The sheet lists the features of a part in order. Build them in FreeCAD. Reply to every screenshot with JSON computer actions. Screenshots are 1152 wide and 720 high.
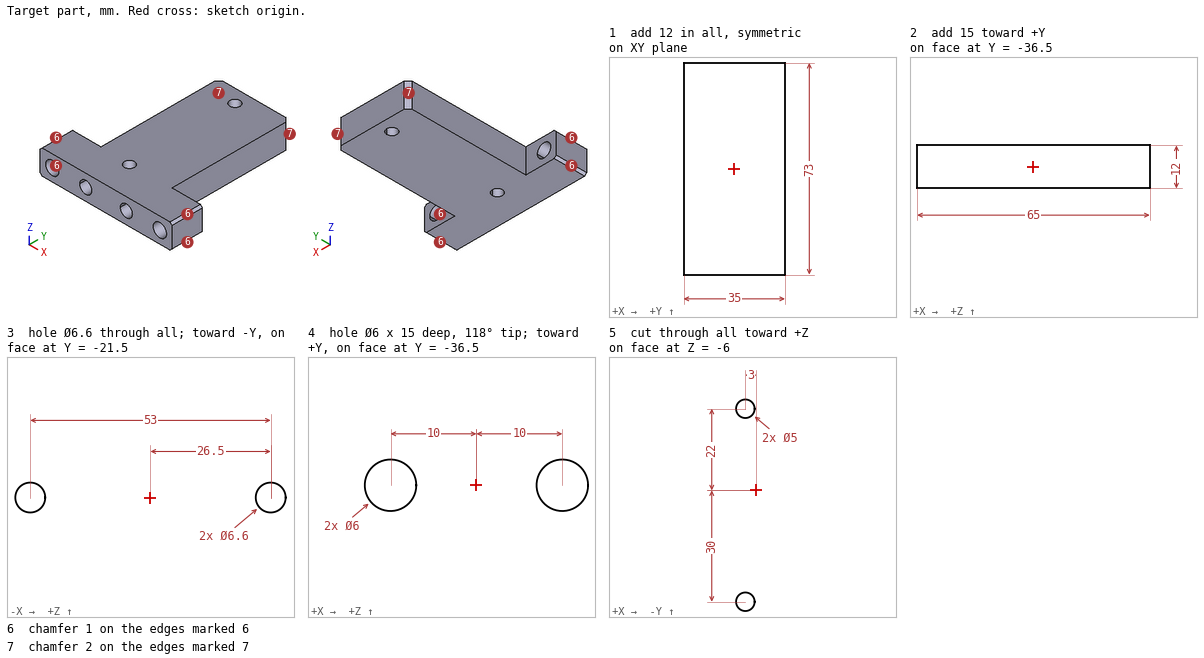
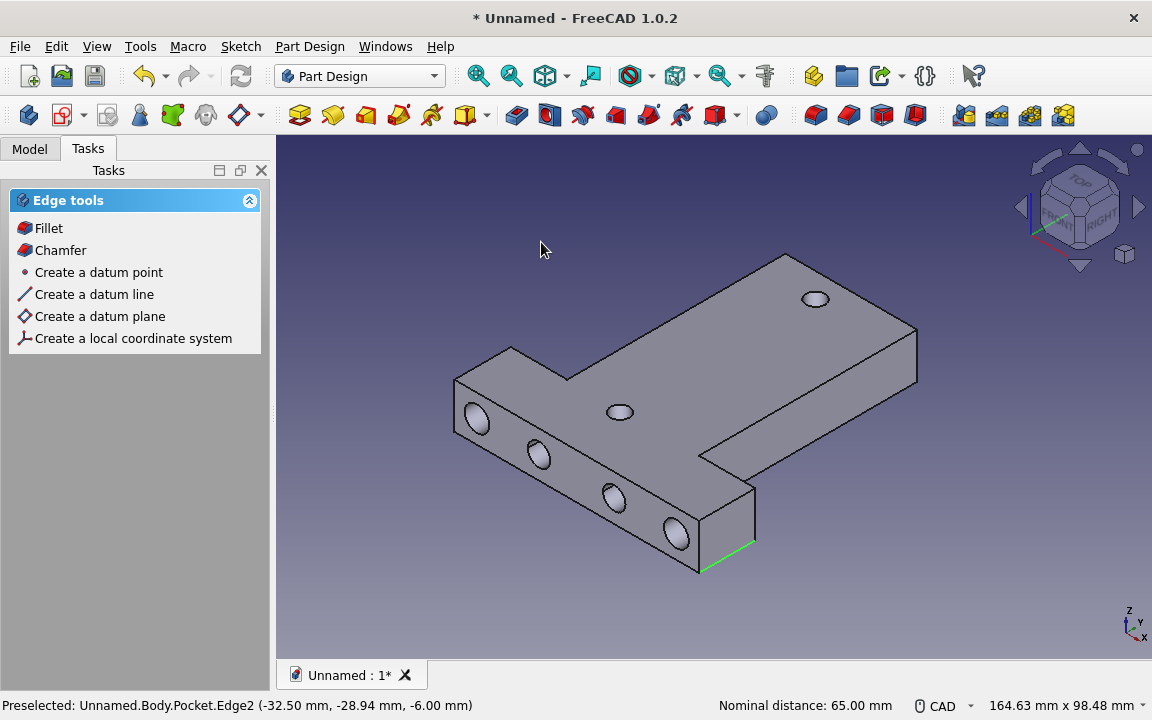
{"action": "left_click", "coordinate": [727, 504], "text": "ctrl"}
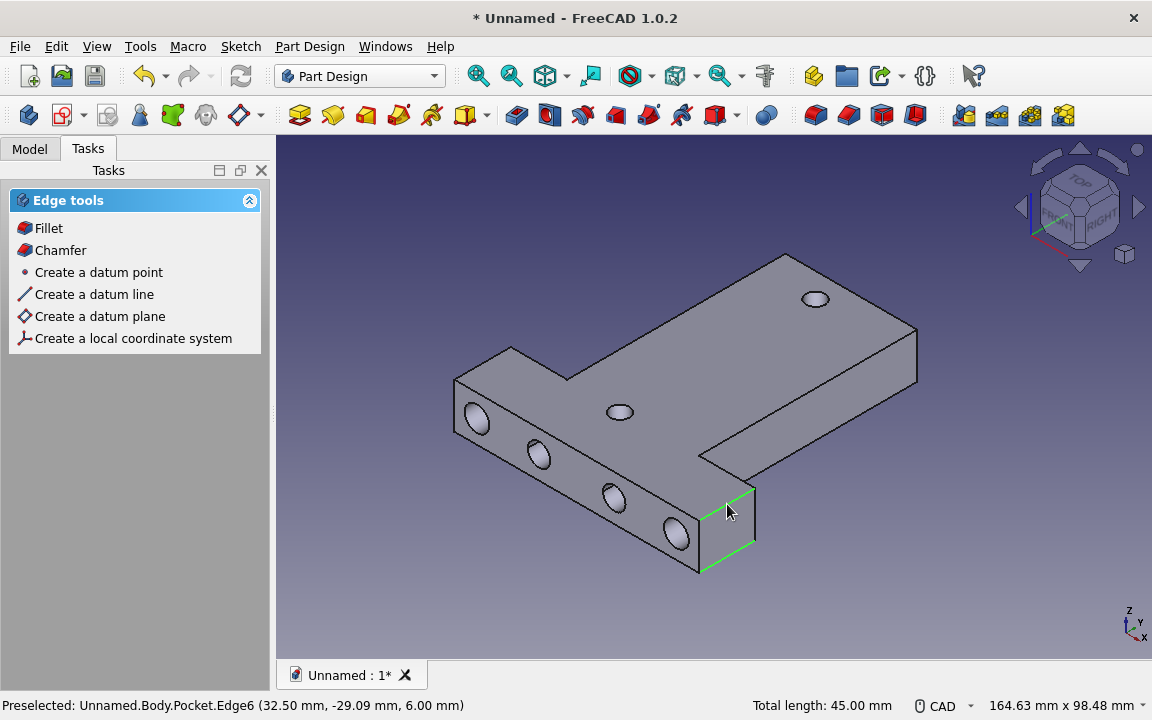
{"action": "key", "text": "2"}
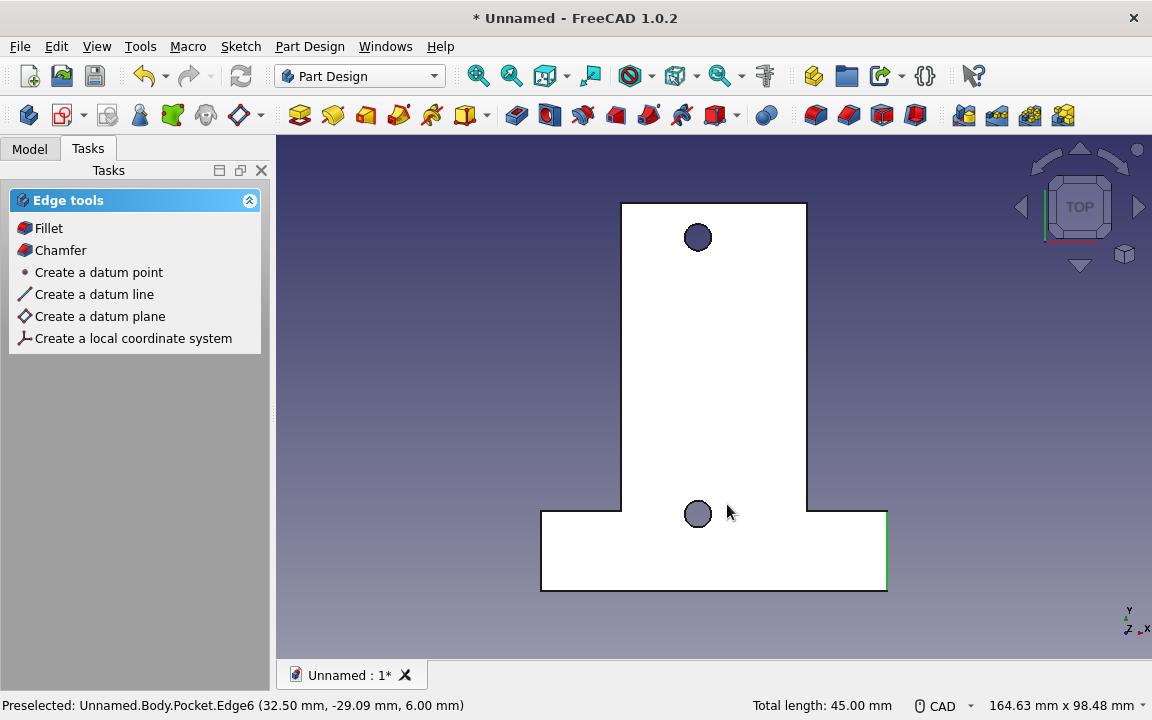
{"action": "left_click", "coordinate": [541, 550], "text": "ctrl"}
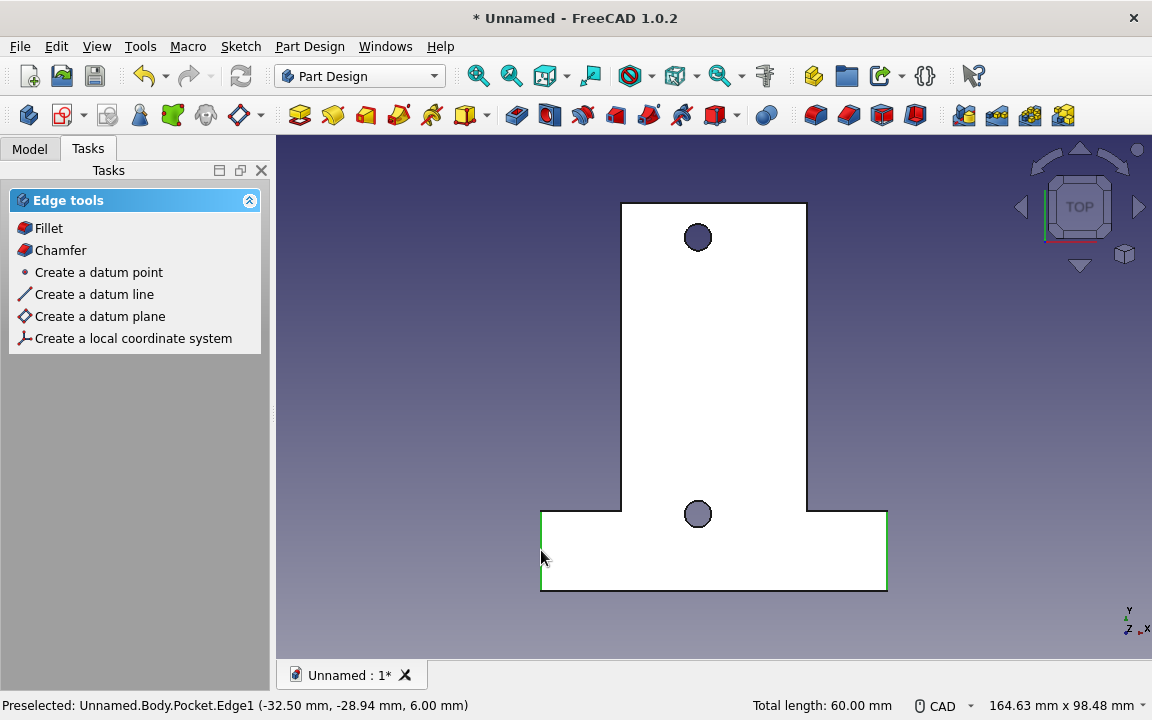
{"action": "left_click", "coordinate": [849, 116]}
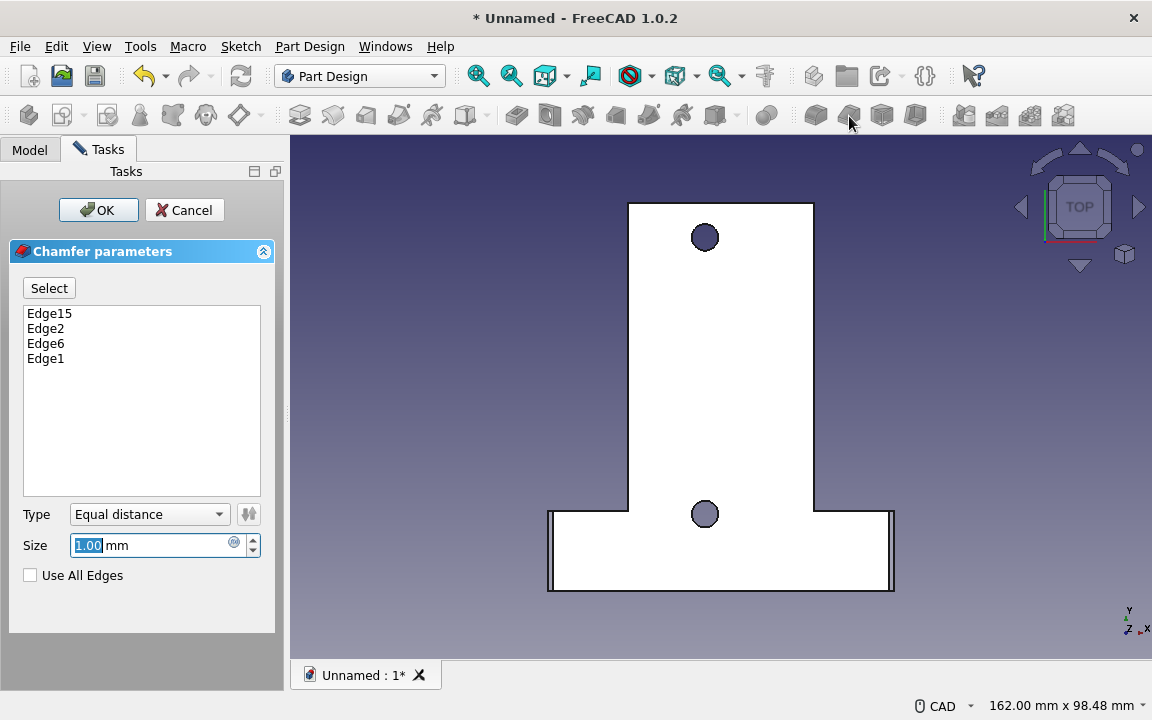
{"action": "type", "text": "1"}
{"action": "key", "text": "Tab"}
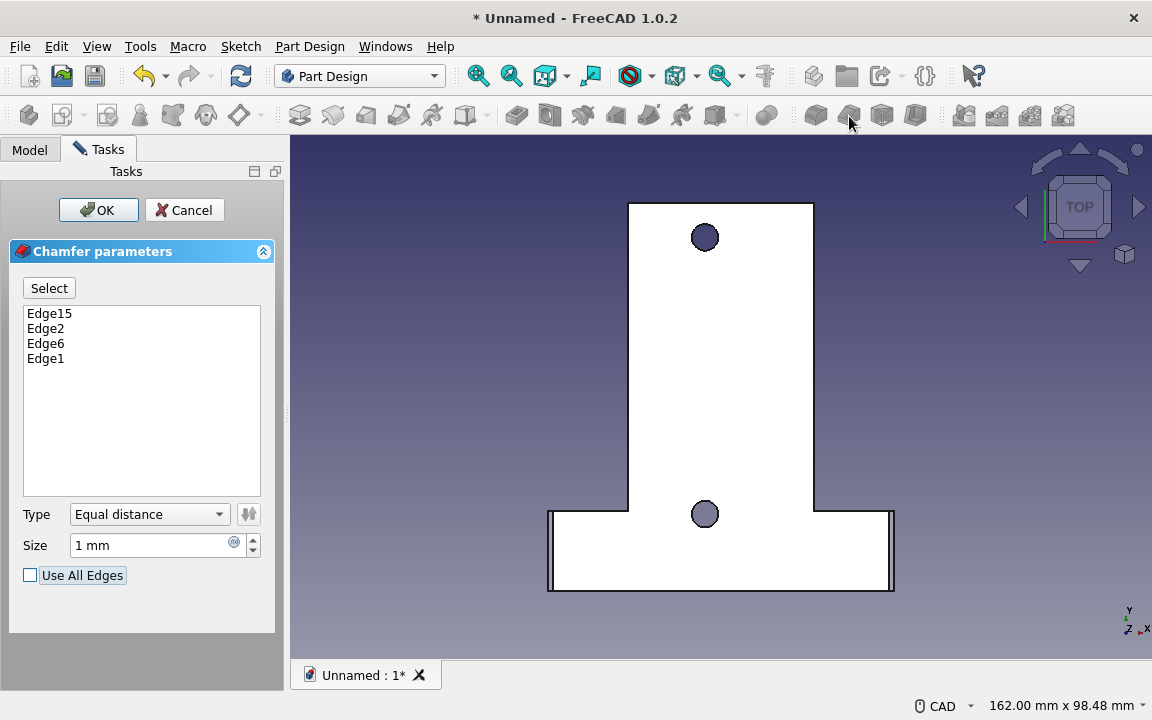
{"action": "left_click", "coordinate": [99, 210]}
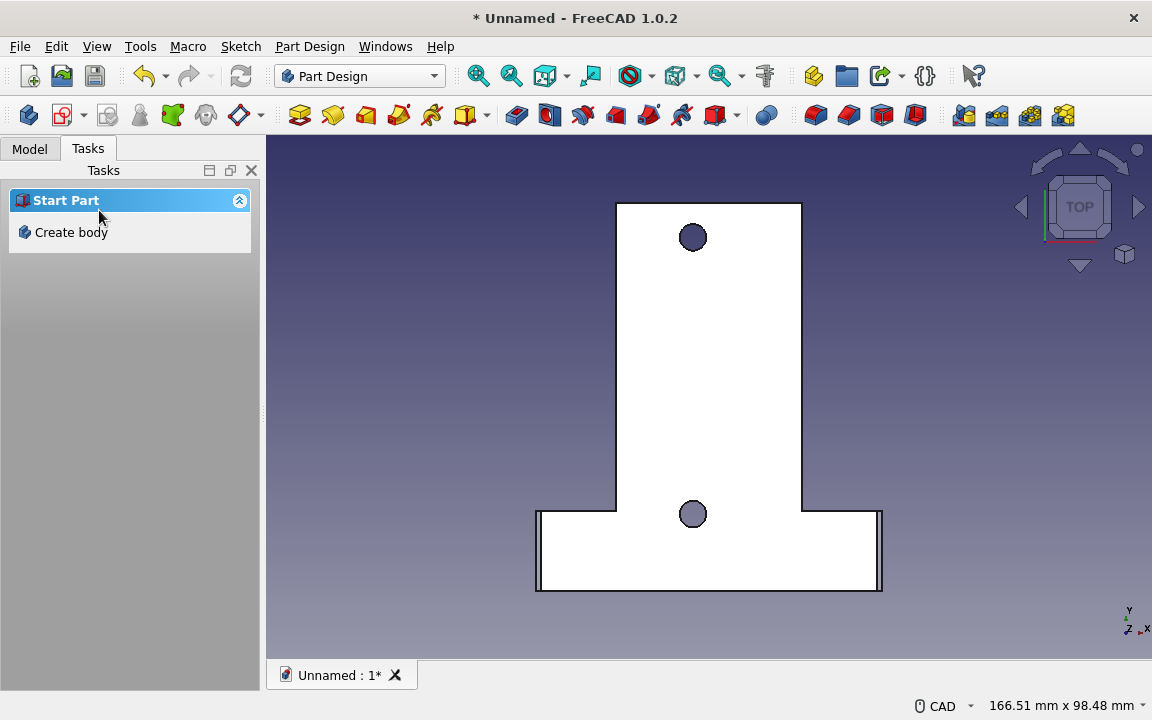
{"action": "key", "text": "0"}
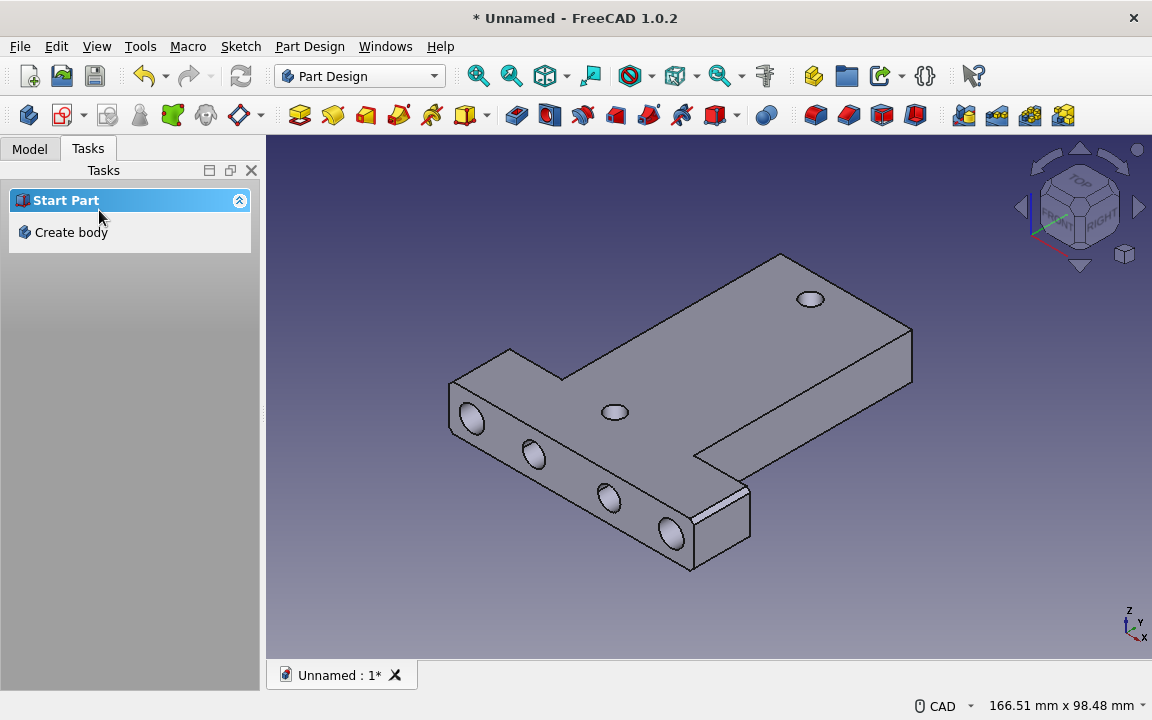
{"action": "key", "text": "2"}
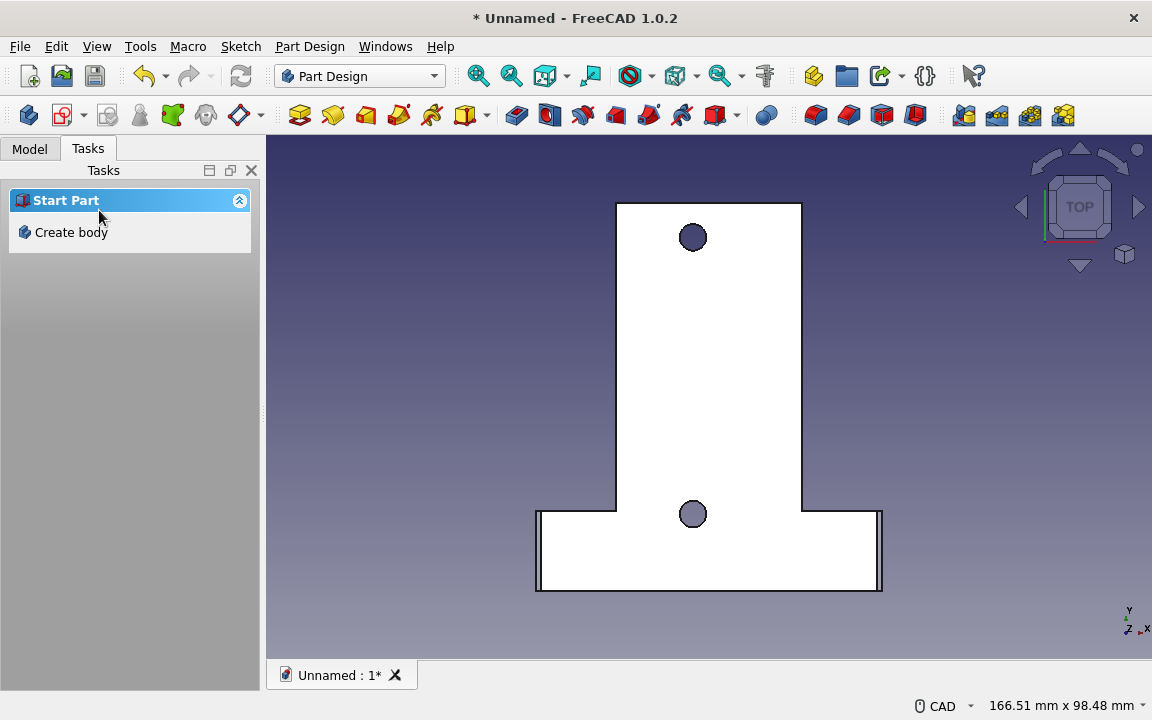
{"action": "key", "text": "1"}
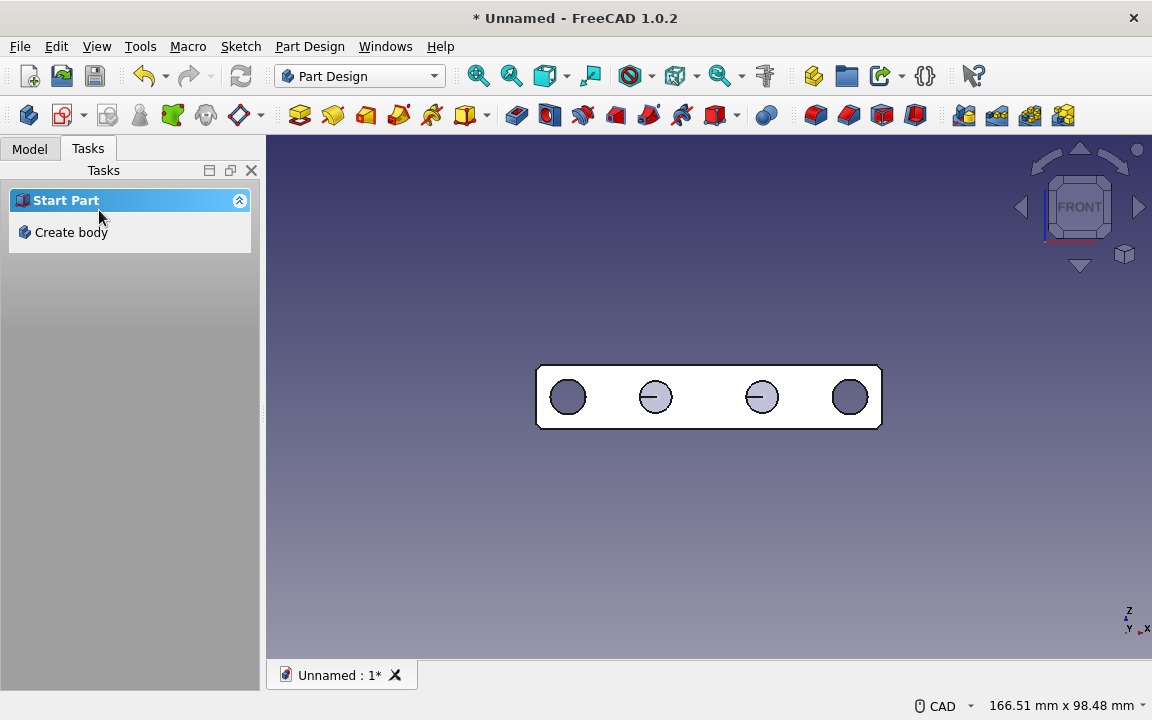
{"action": "left_click", "coordinate": [479, 76]}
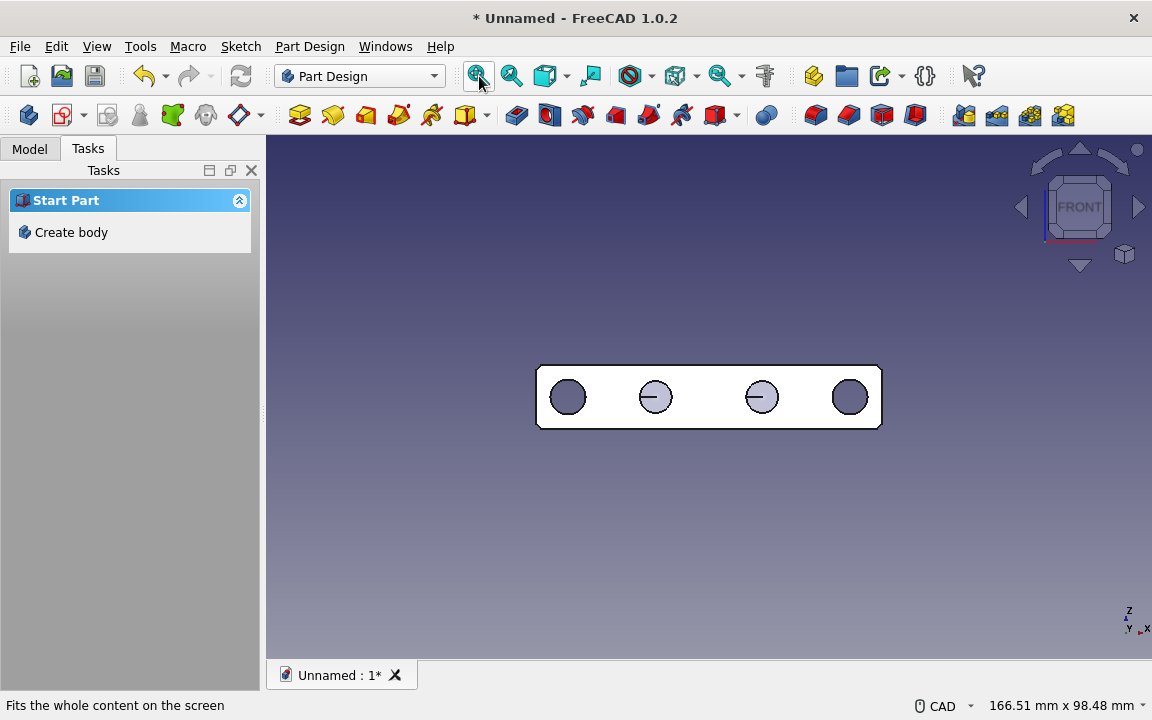
{"action": "key", "text": "3"}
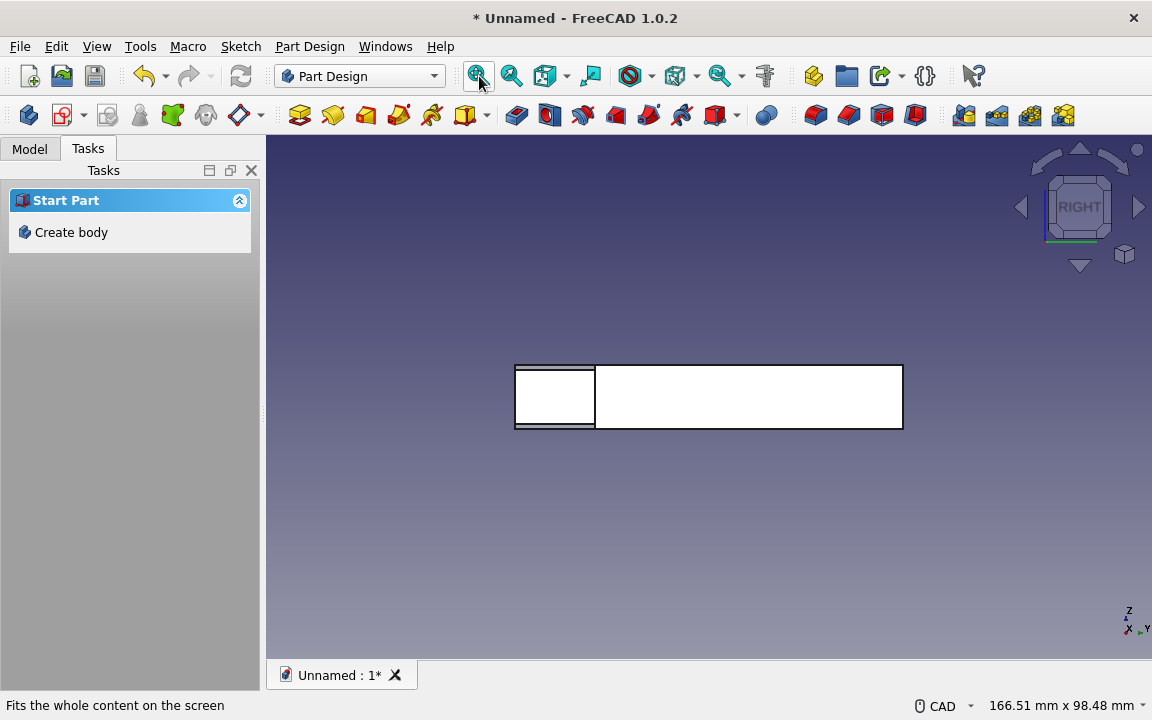
{"action": "left_click", "coordinate": [479, 76]}